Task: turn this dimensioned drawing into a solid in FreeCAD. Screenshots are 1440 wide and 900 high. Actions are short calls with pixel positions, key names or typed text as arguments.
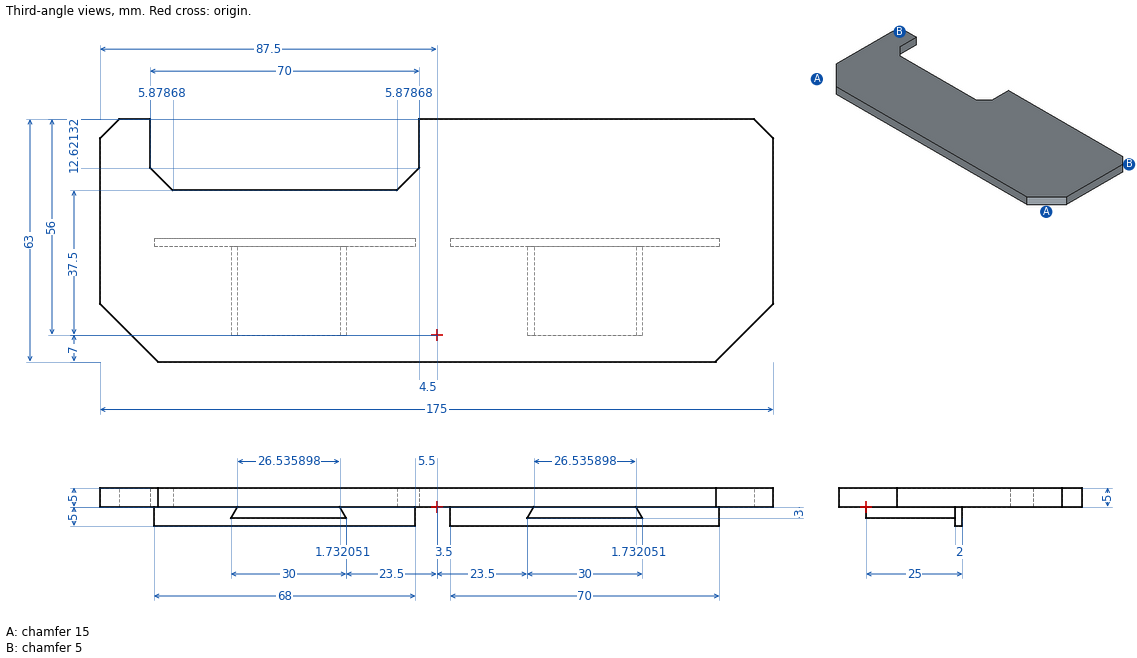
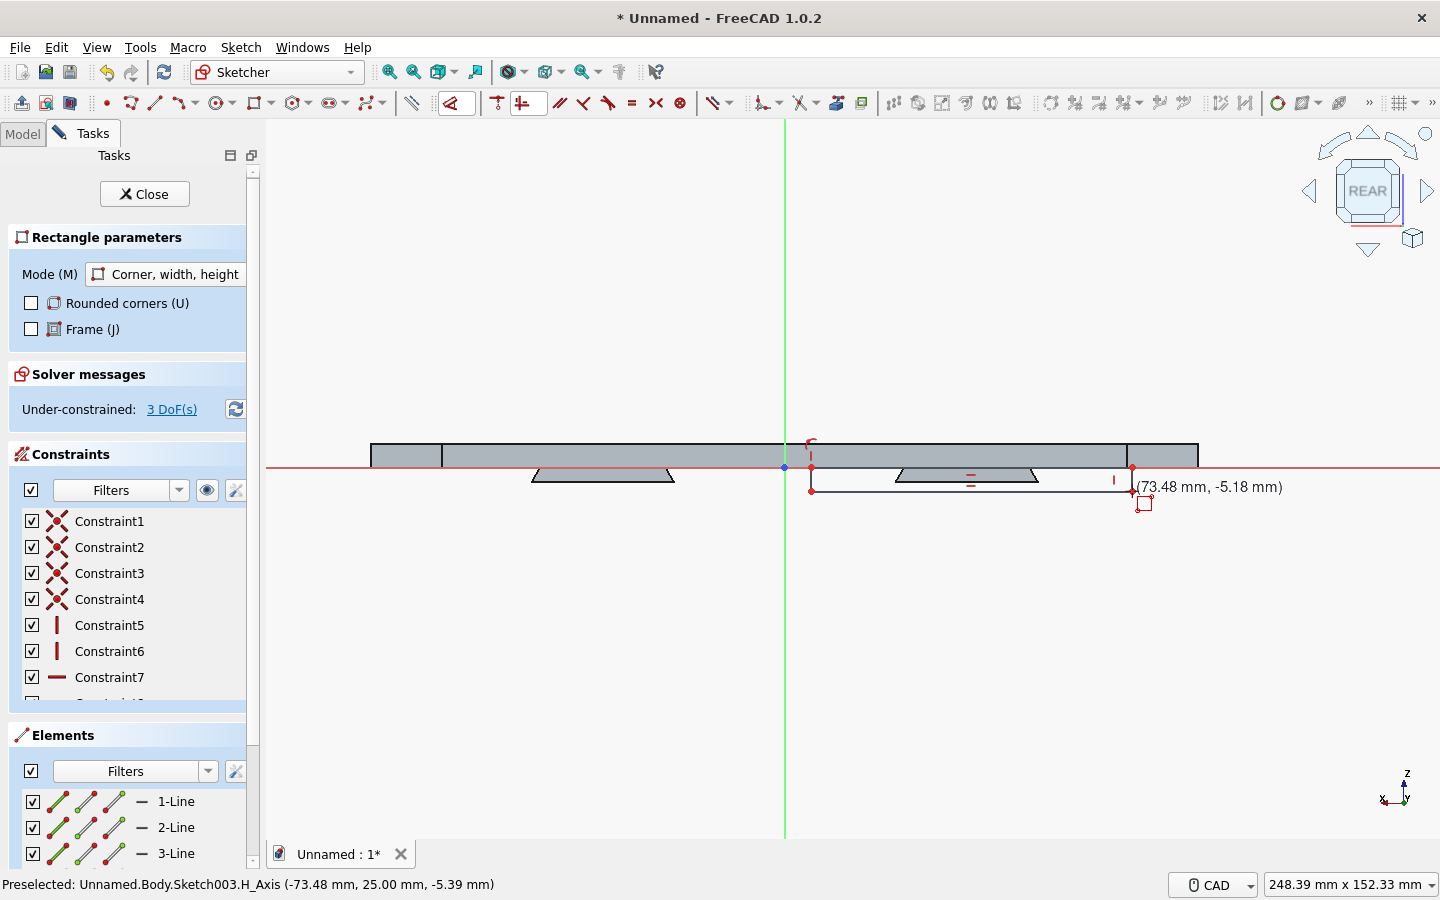
click(437, 468)
click(768, 491)
key(Escape)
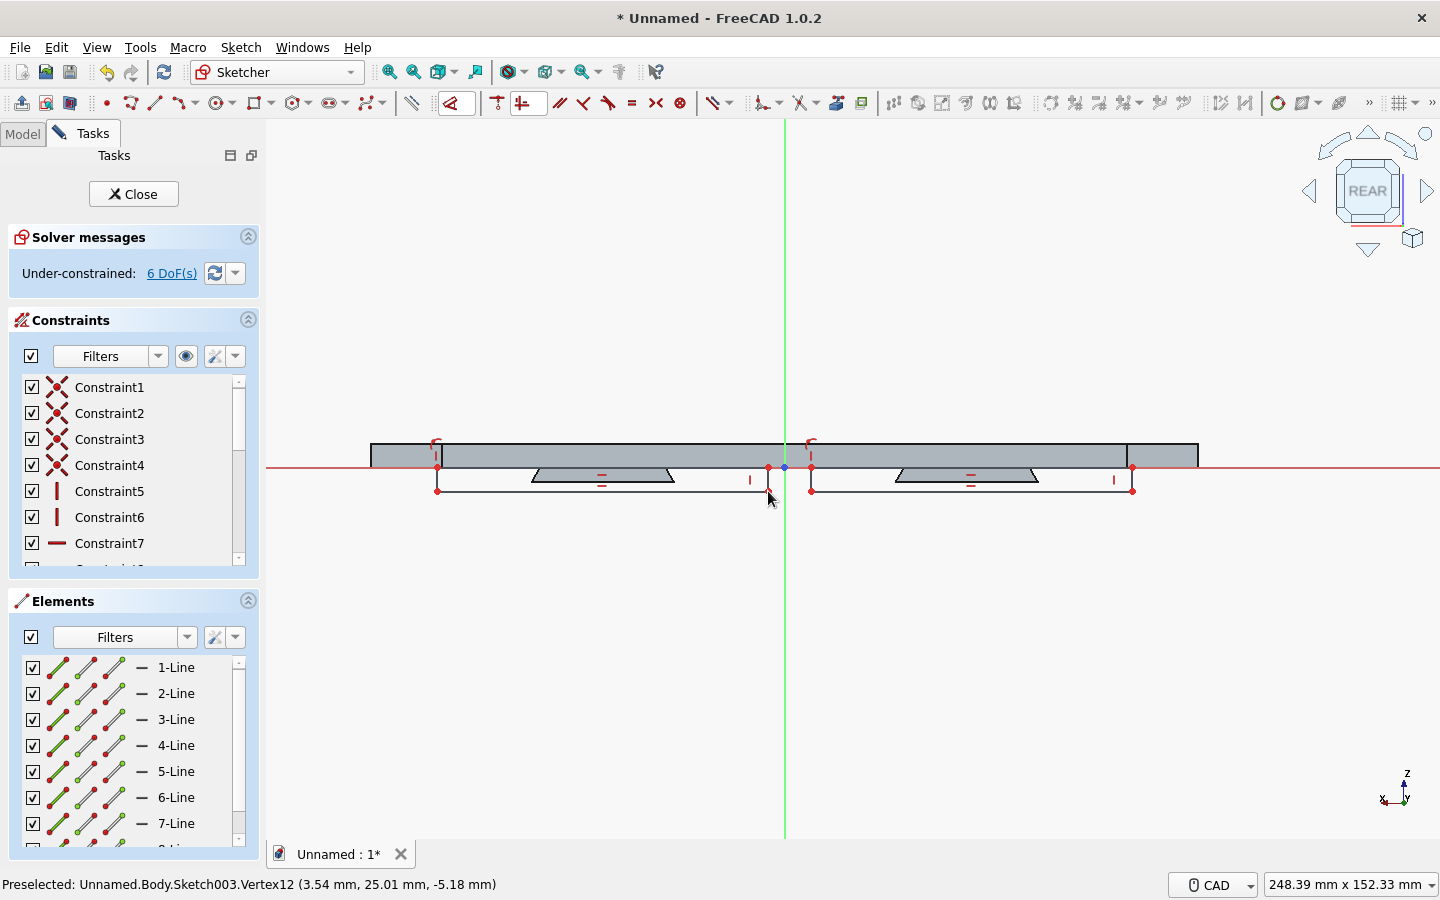
scroll(811, 477, up, 3)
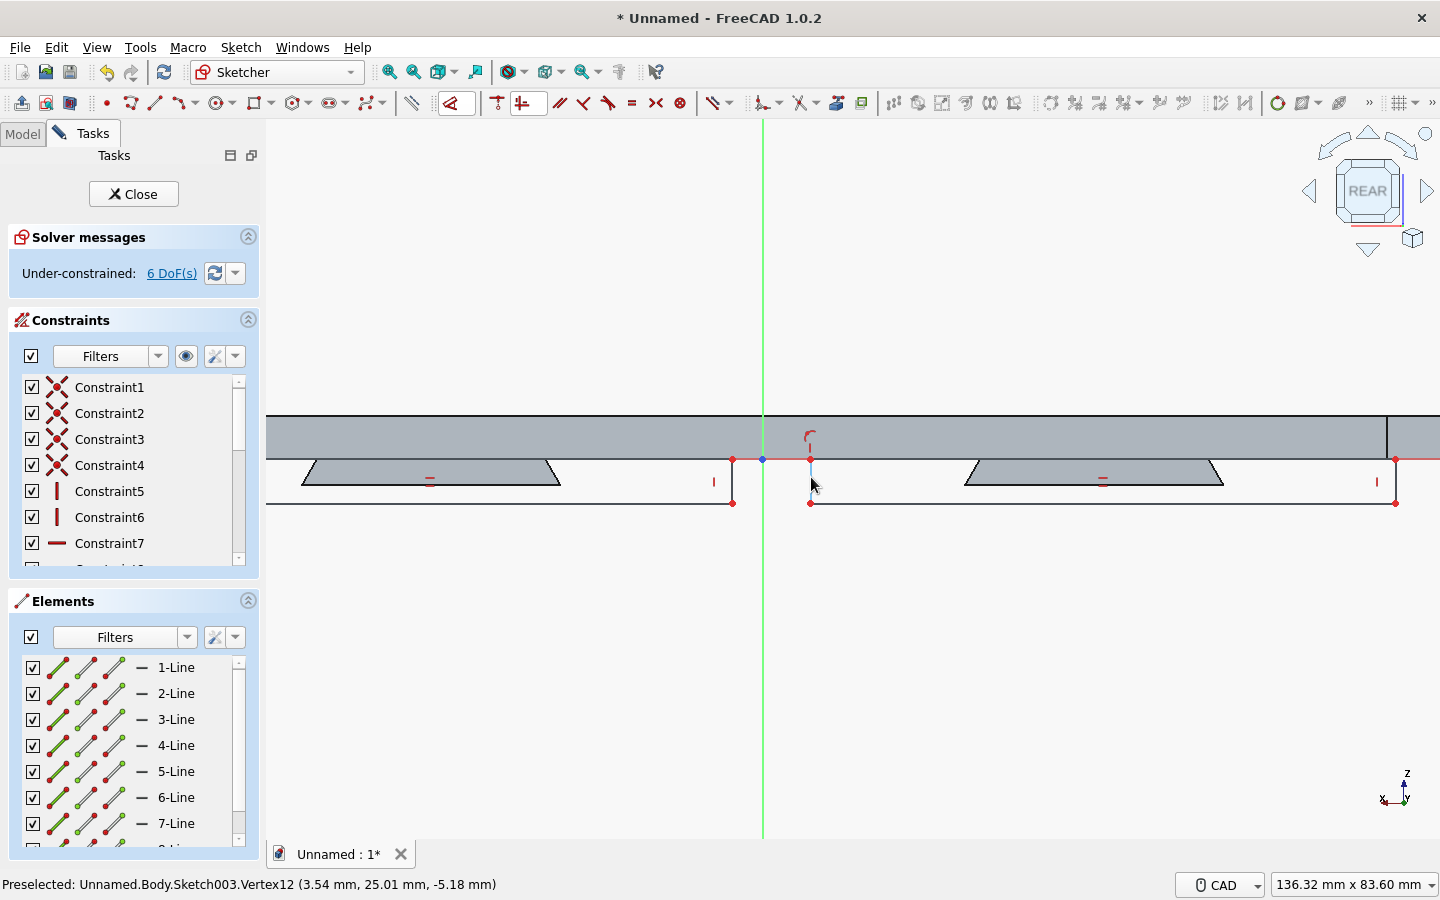
click(811, 477)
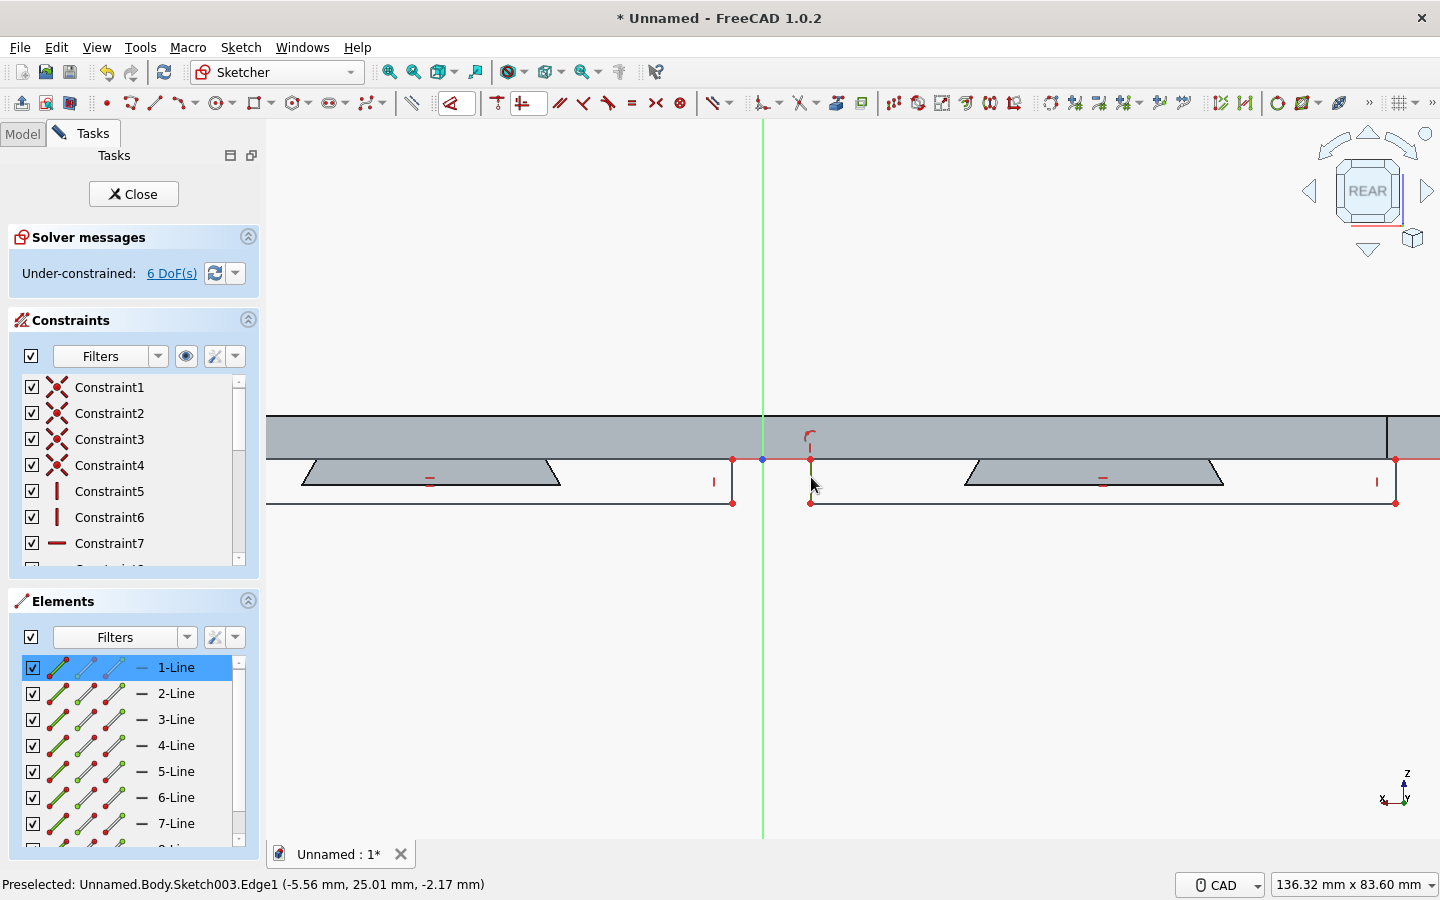
click(470, 104)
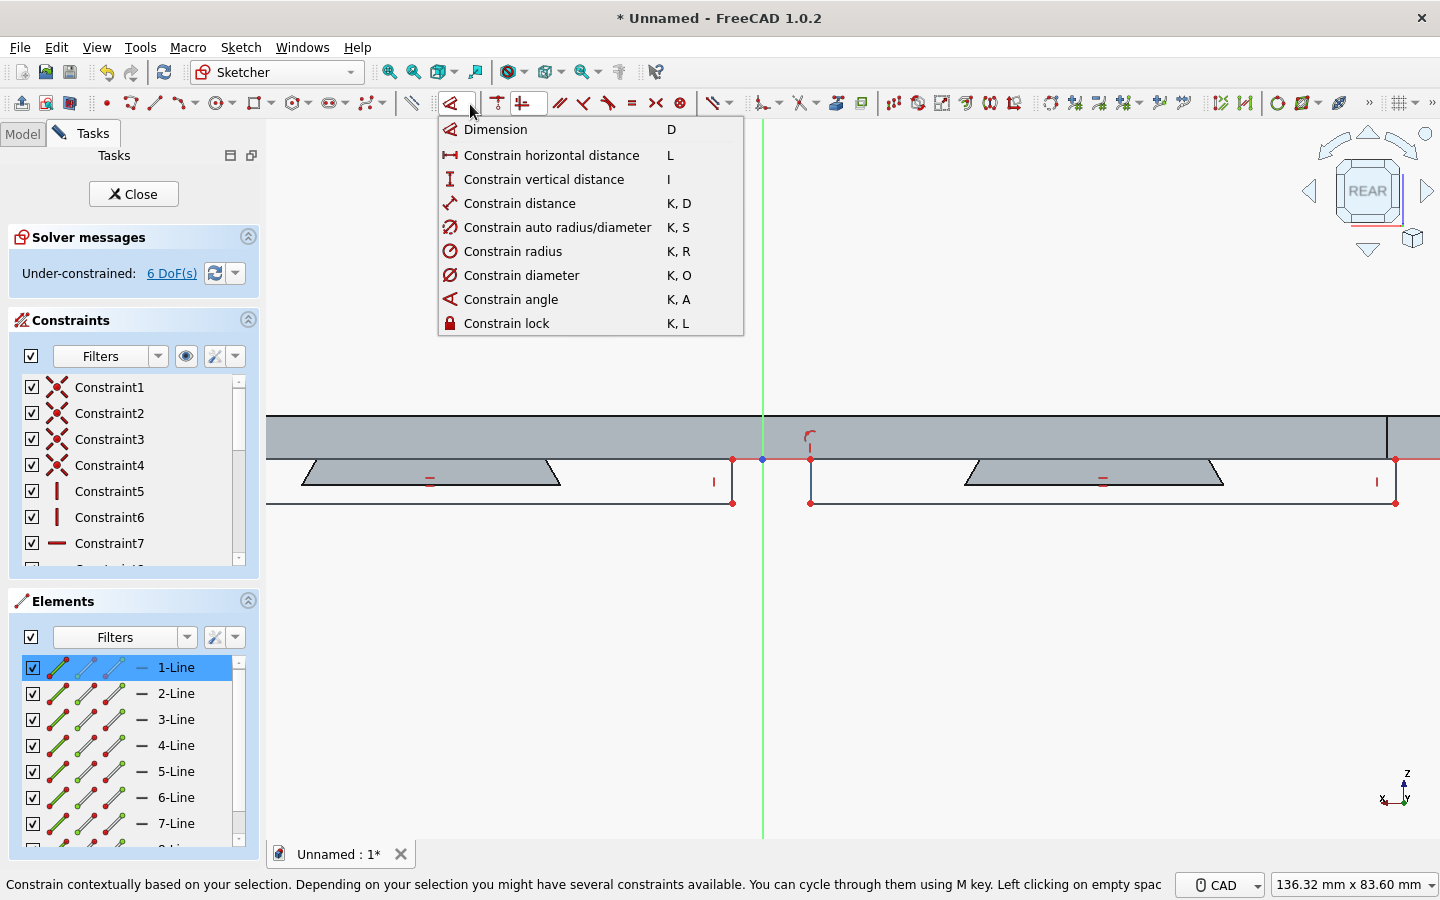
click(591, 179)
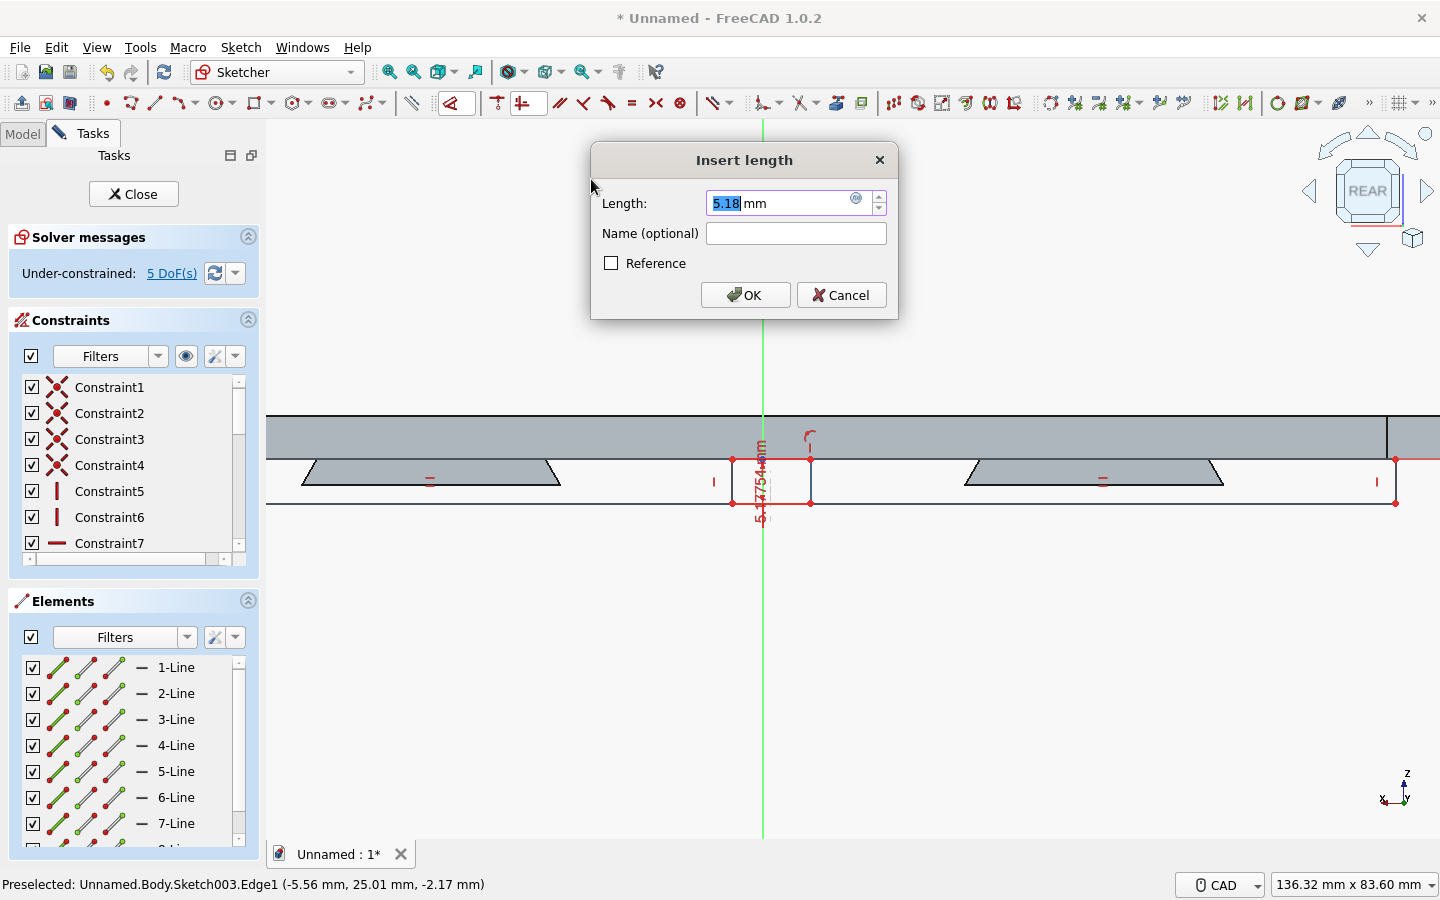
text(5)
key(Return)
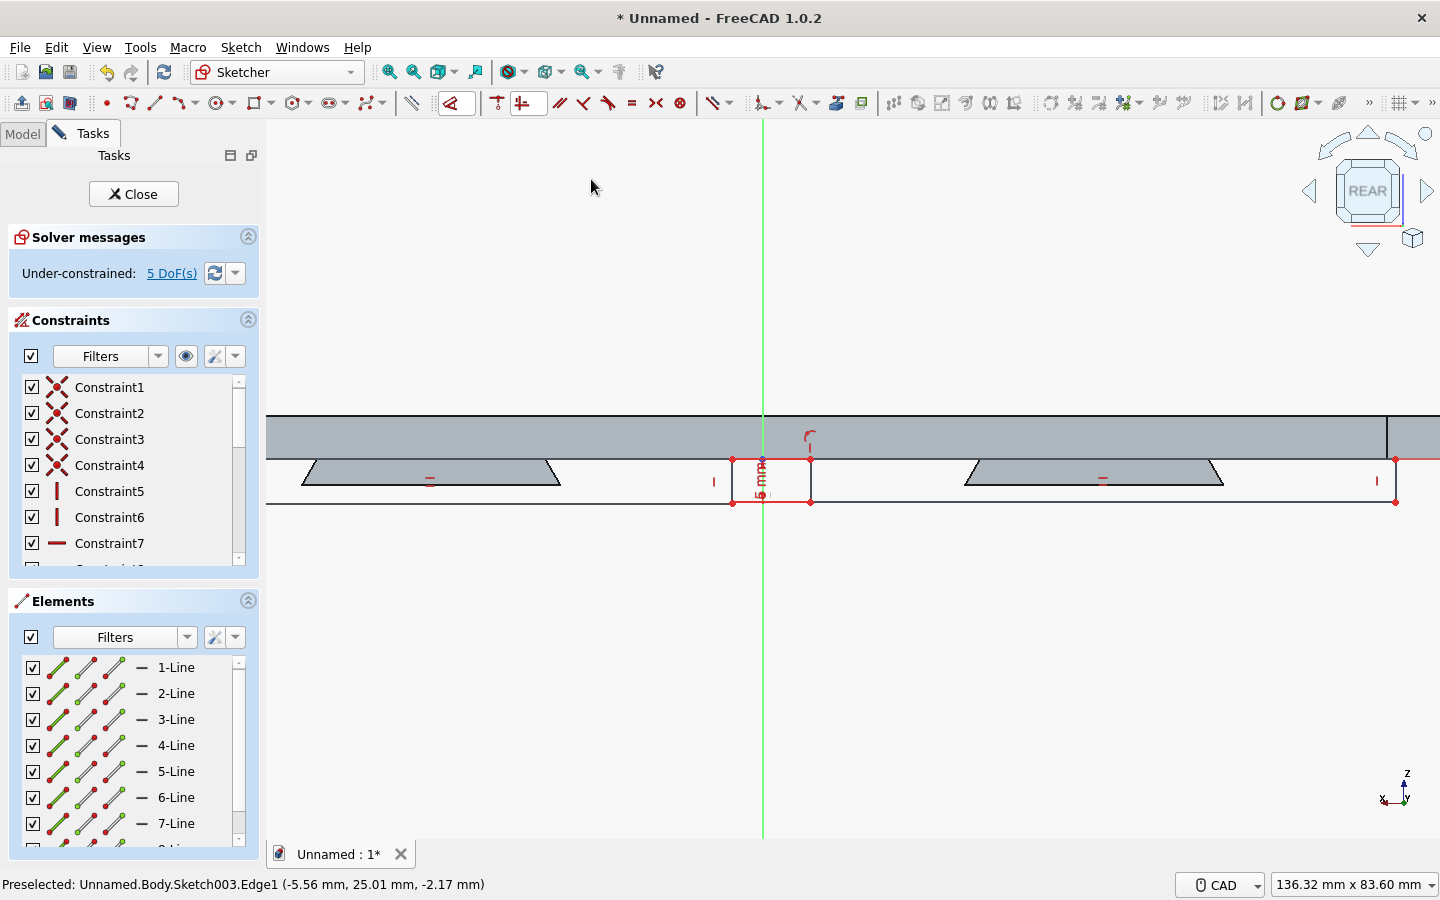
scroll(811, 477, down, 3)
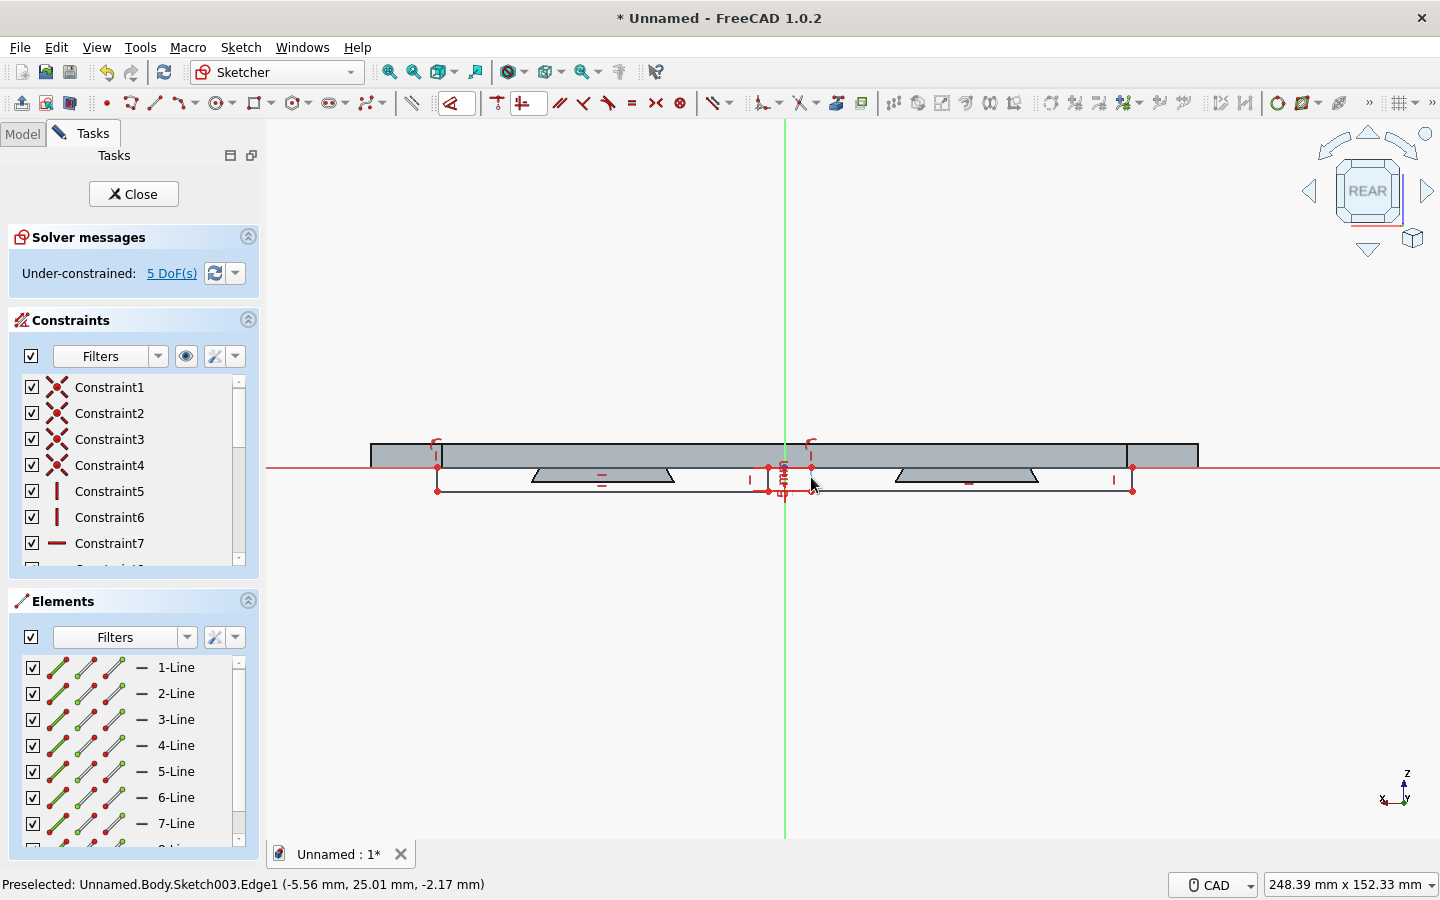
scroll(437, 475, up, 4)